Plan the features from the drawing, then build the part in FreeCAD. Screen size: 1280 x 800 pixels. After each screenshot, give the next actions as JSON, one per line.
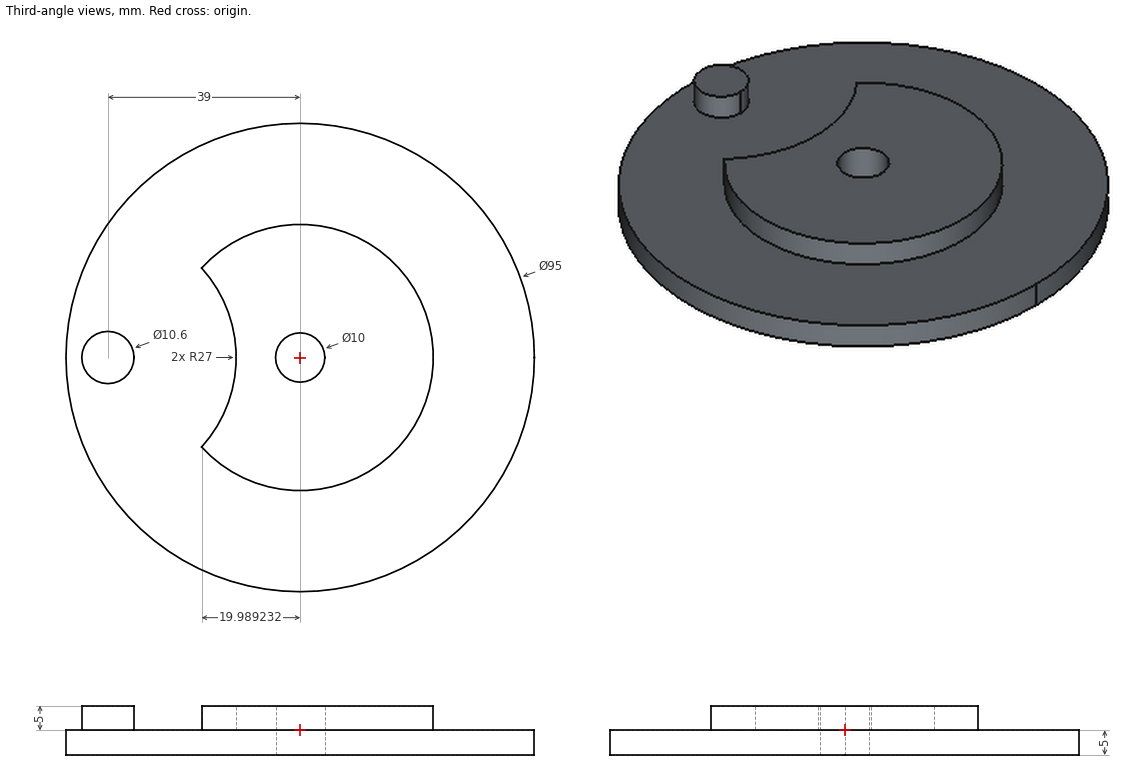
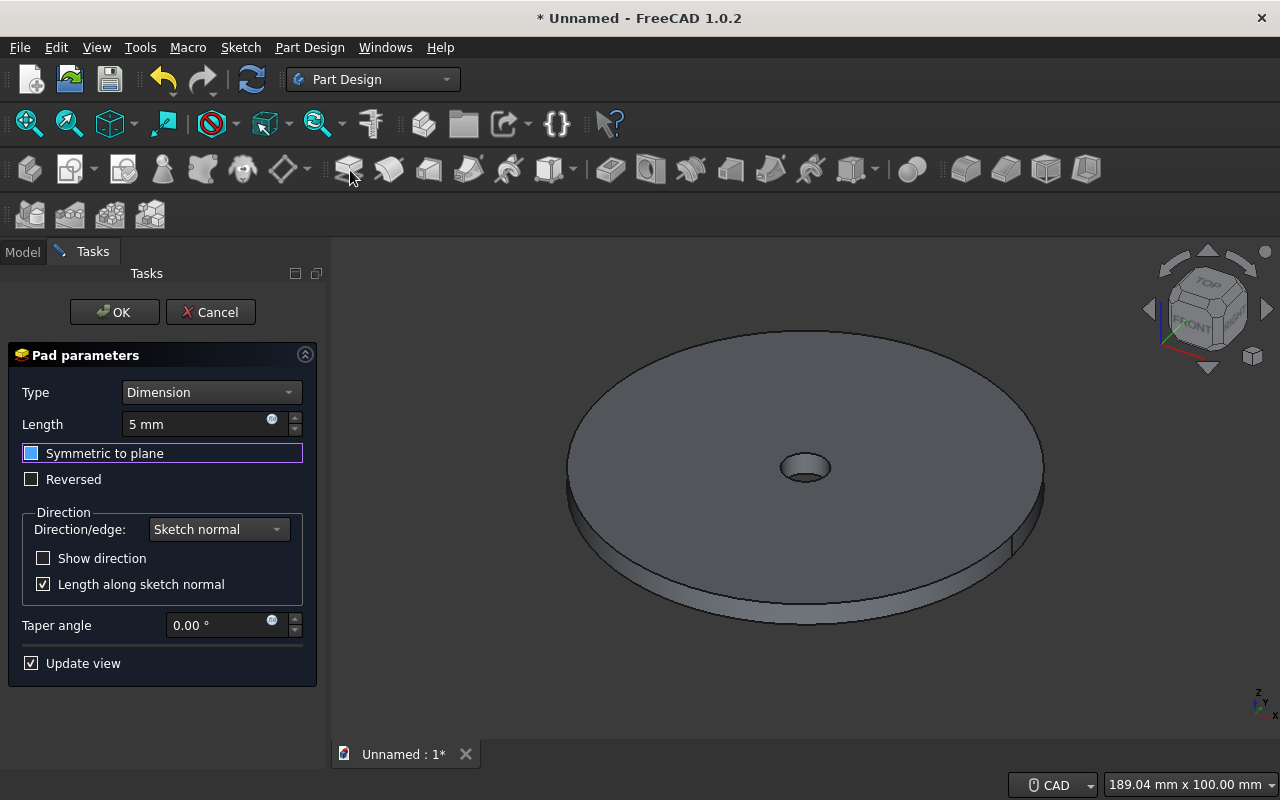
{"action": "left_click", "coordinate": [30, 479]}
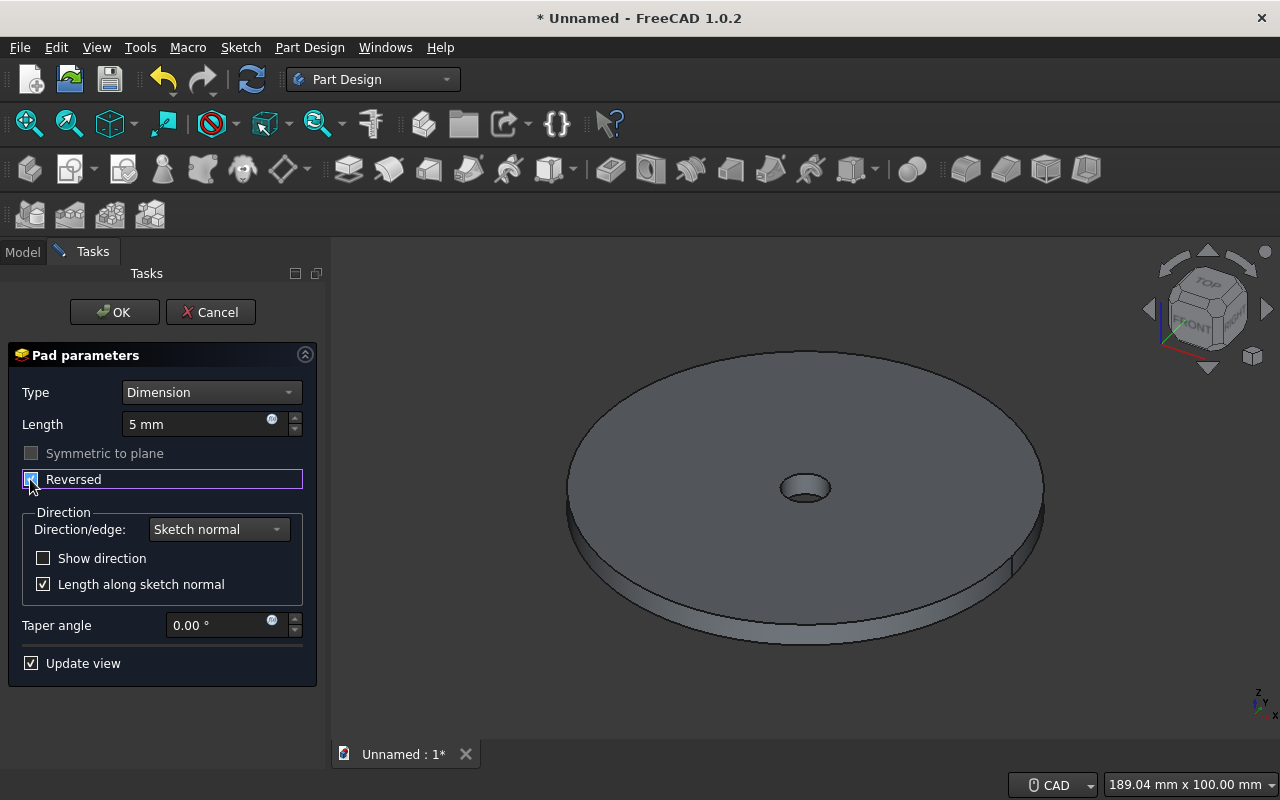
{"action": "left_click", "coordinate": [115, 312]}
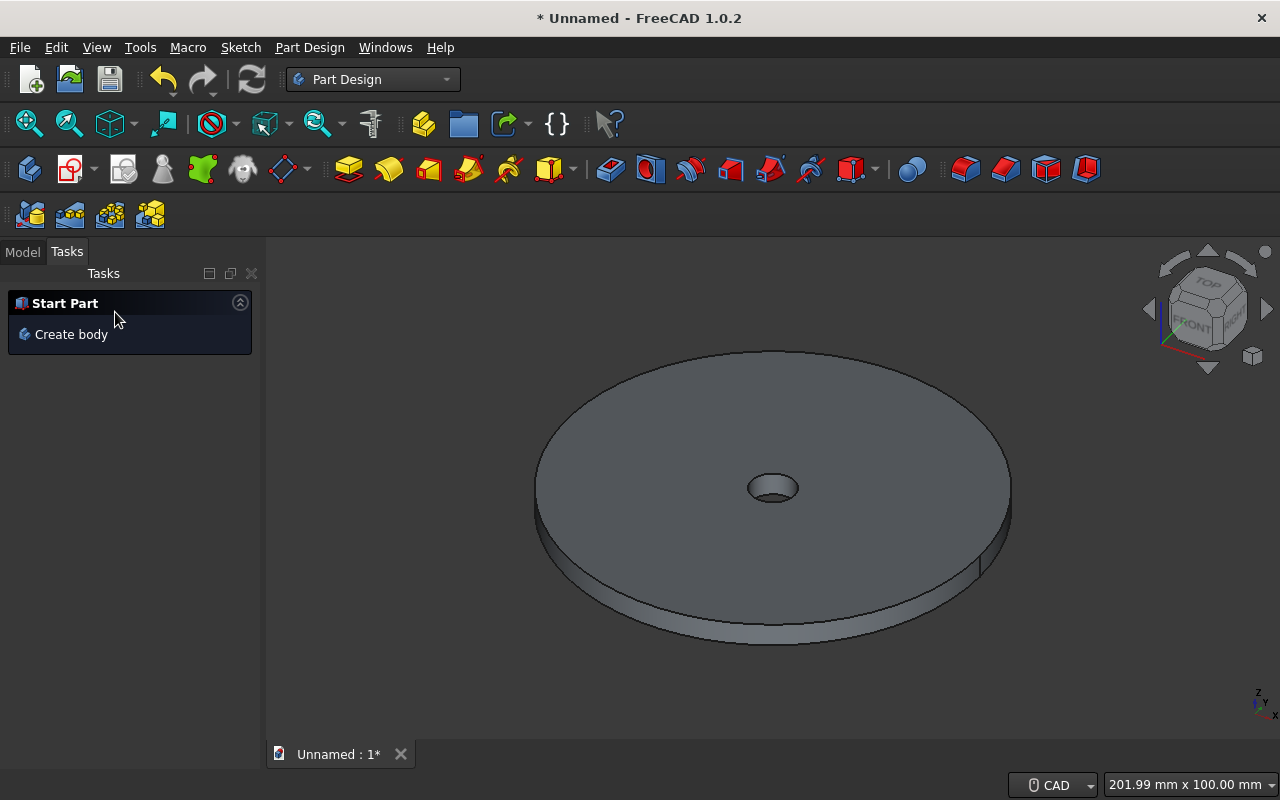
{"action": "left_click", "coordinate": [23, 251]}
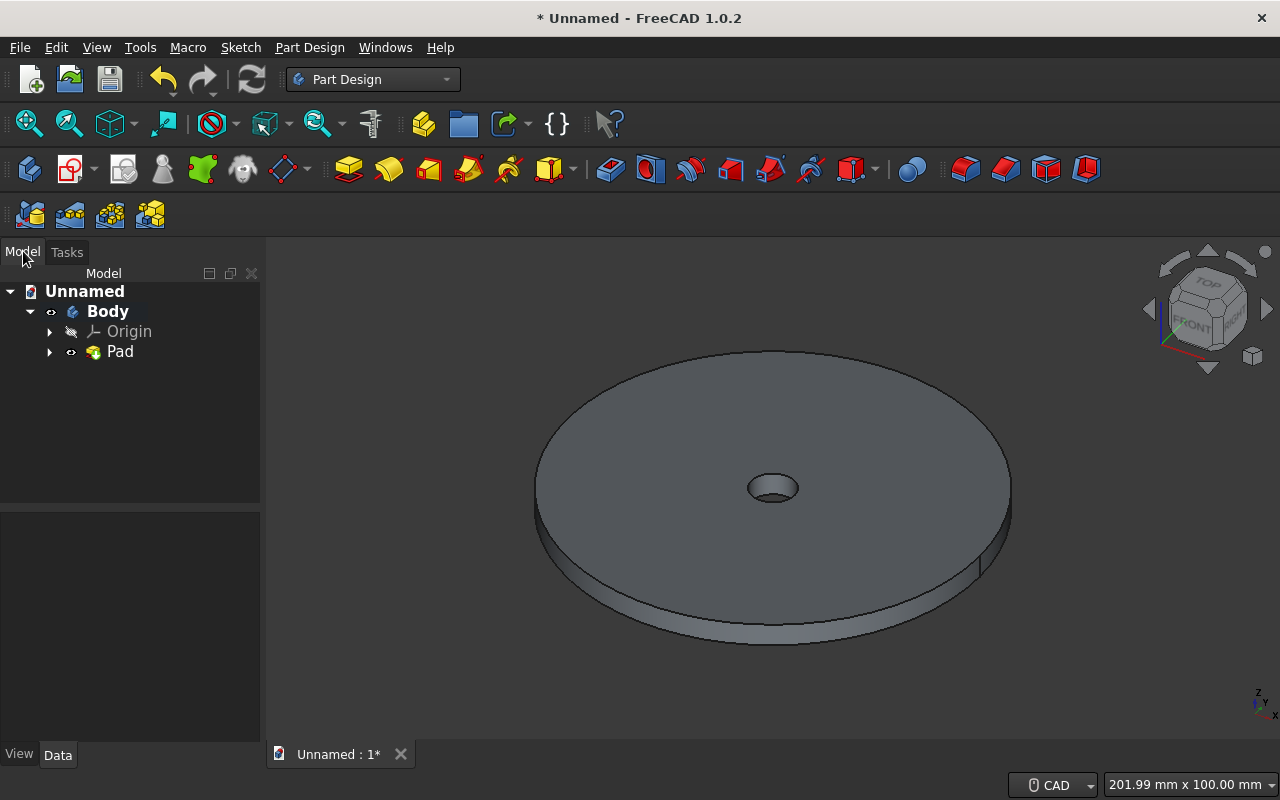
{"action": "left_click", "coordinate": [50, 332]}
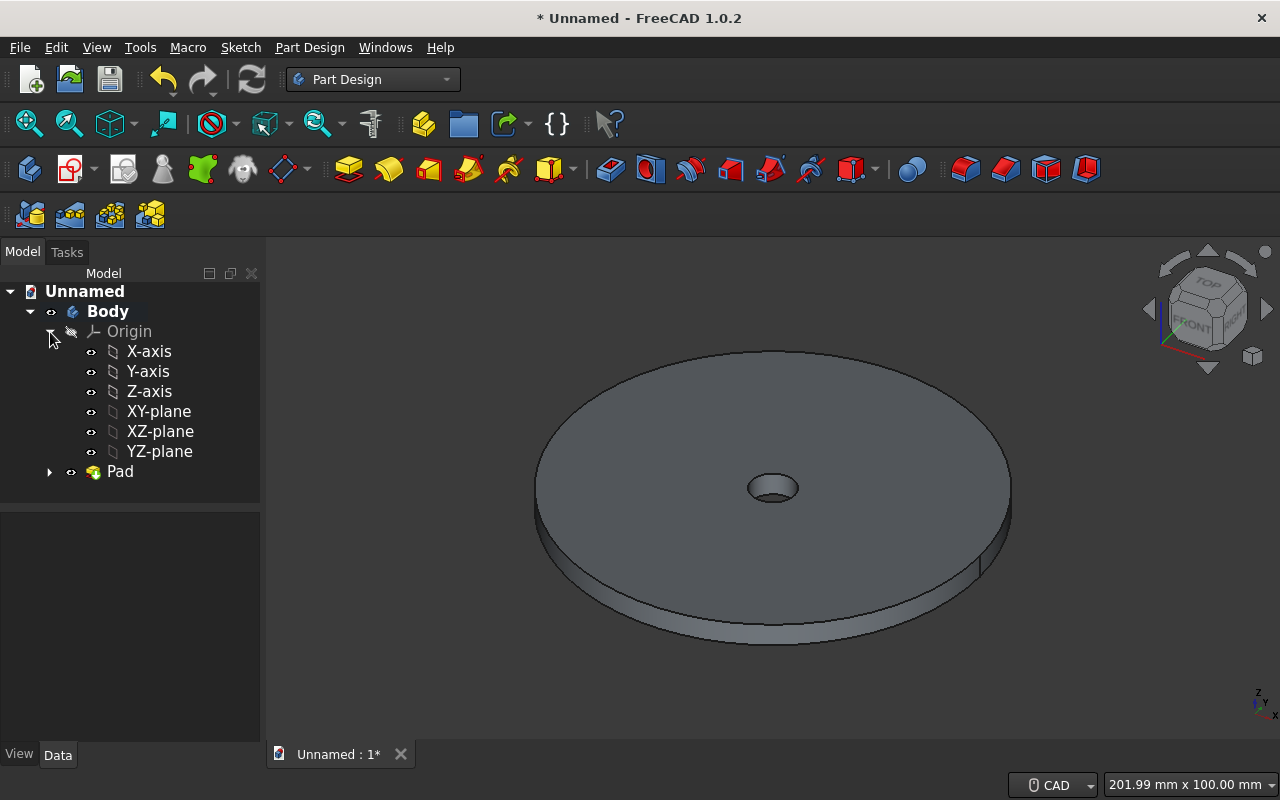
{"action": "left_click", "coordinate": [136, 412]}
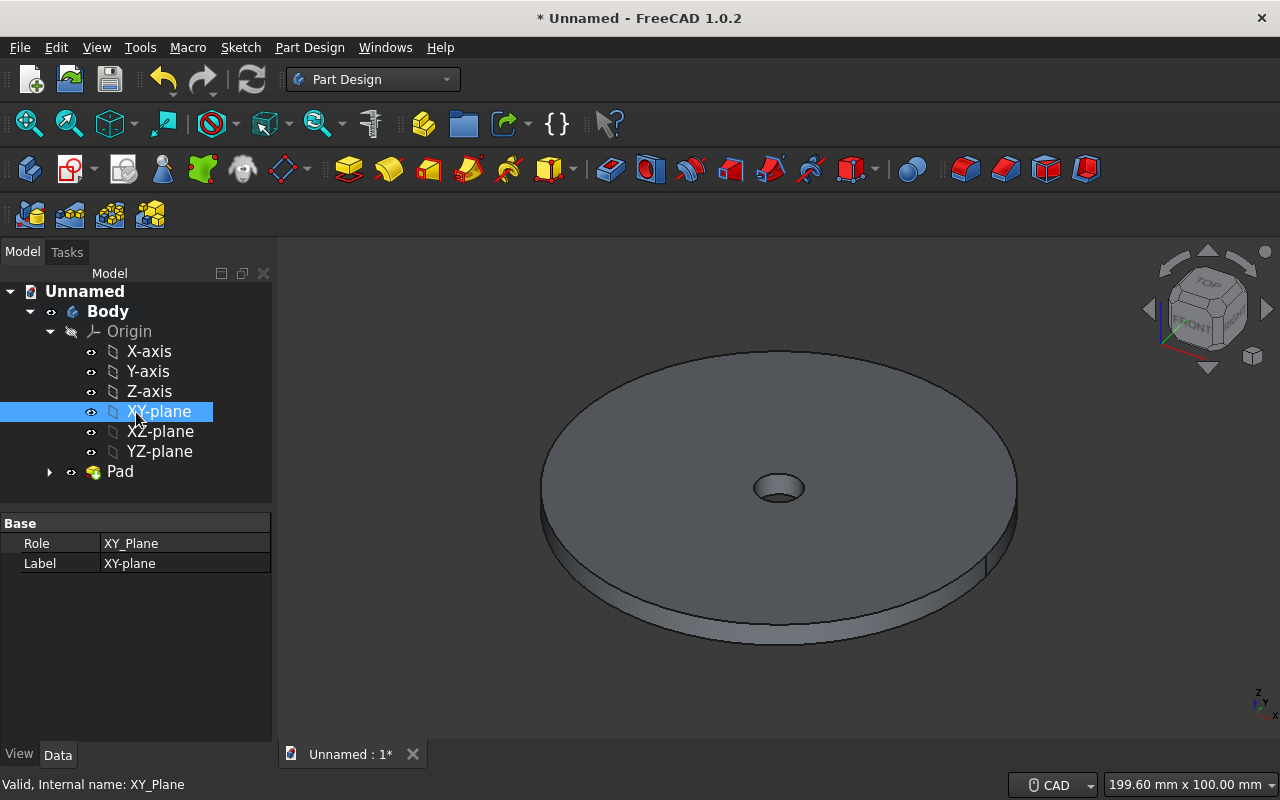
{"action": "left_click", "coordinate": [284, 170]}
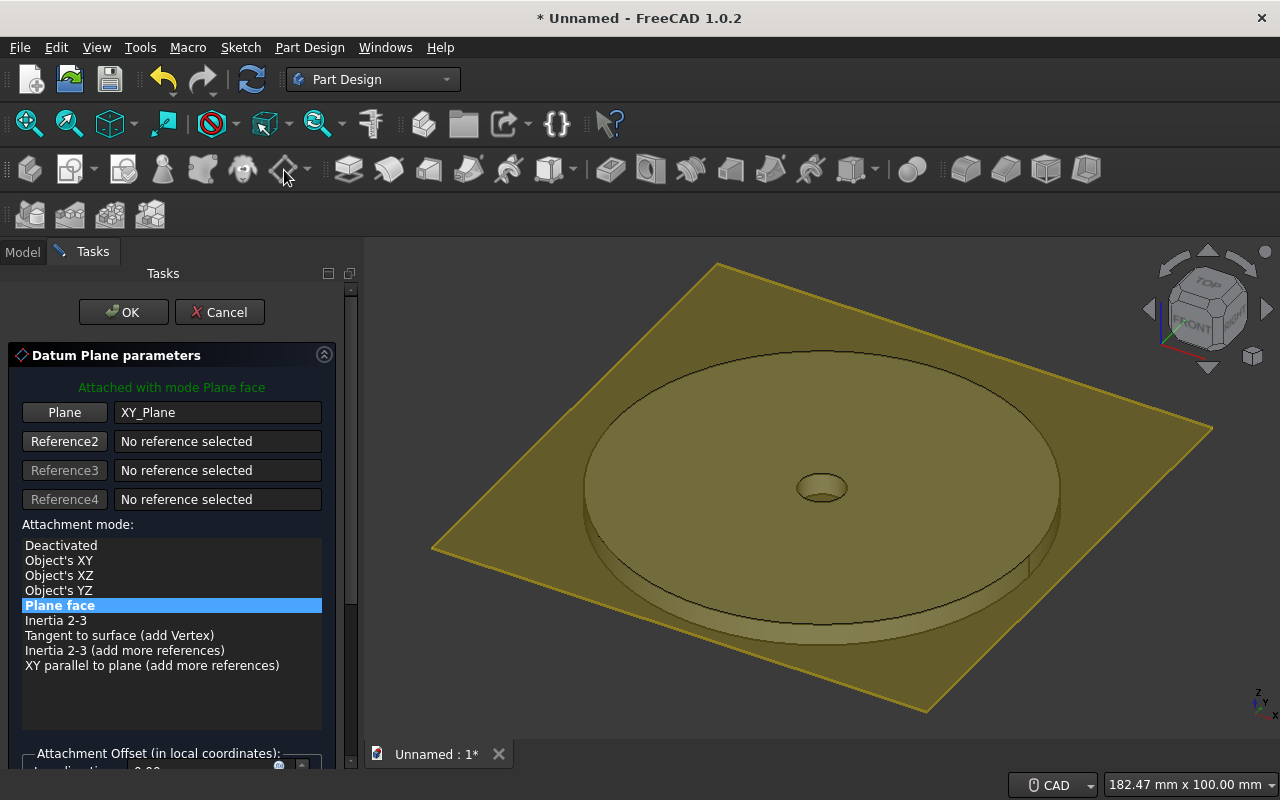
{"action": "scroll", "coordinate": [351, 526], "scroll_direction": "down", "scroll_amount": 3}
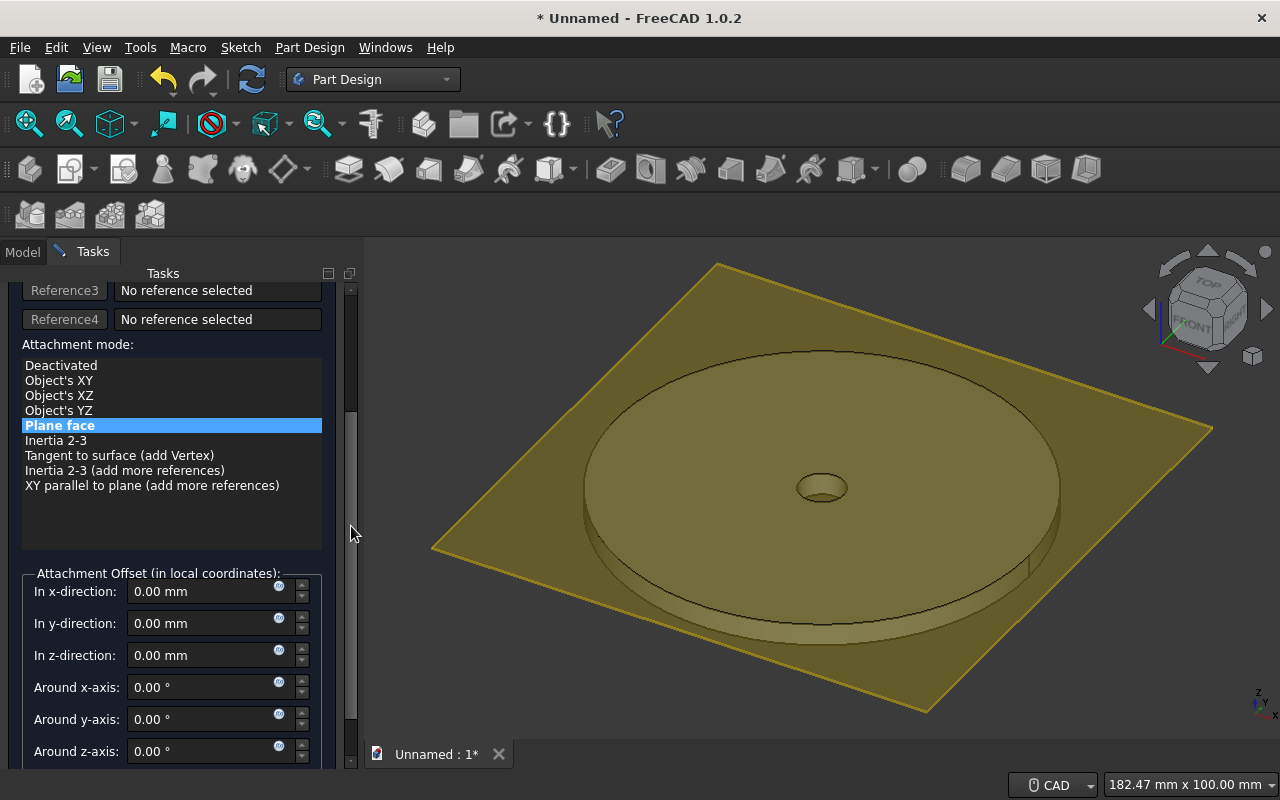
{"action": "triple_click", "coordinate": [210, 655]}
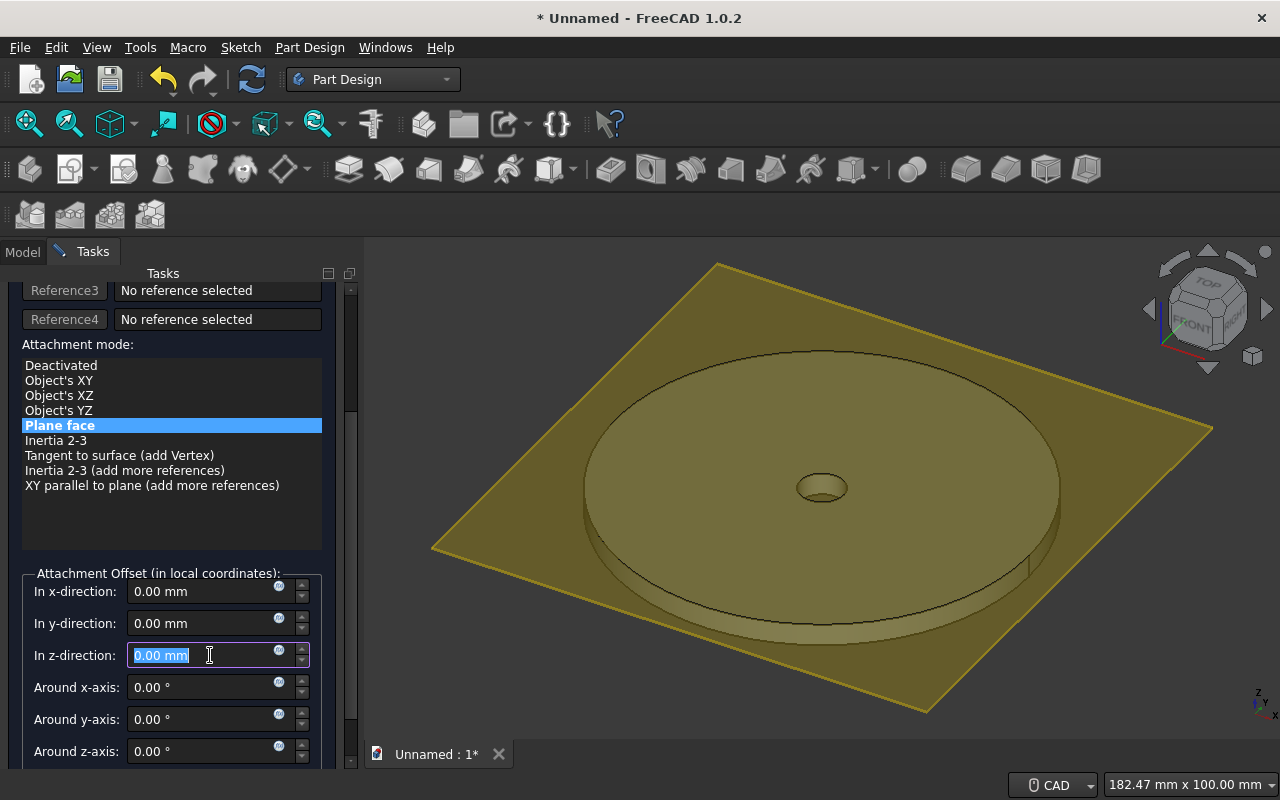
{"action": "type", "text": "5"}
{"action": "key", "text": "Tab"}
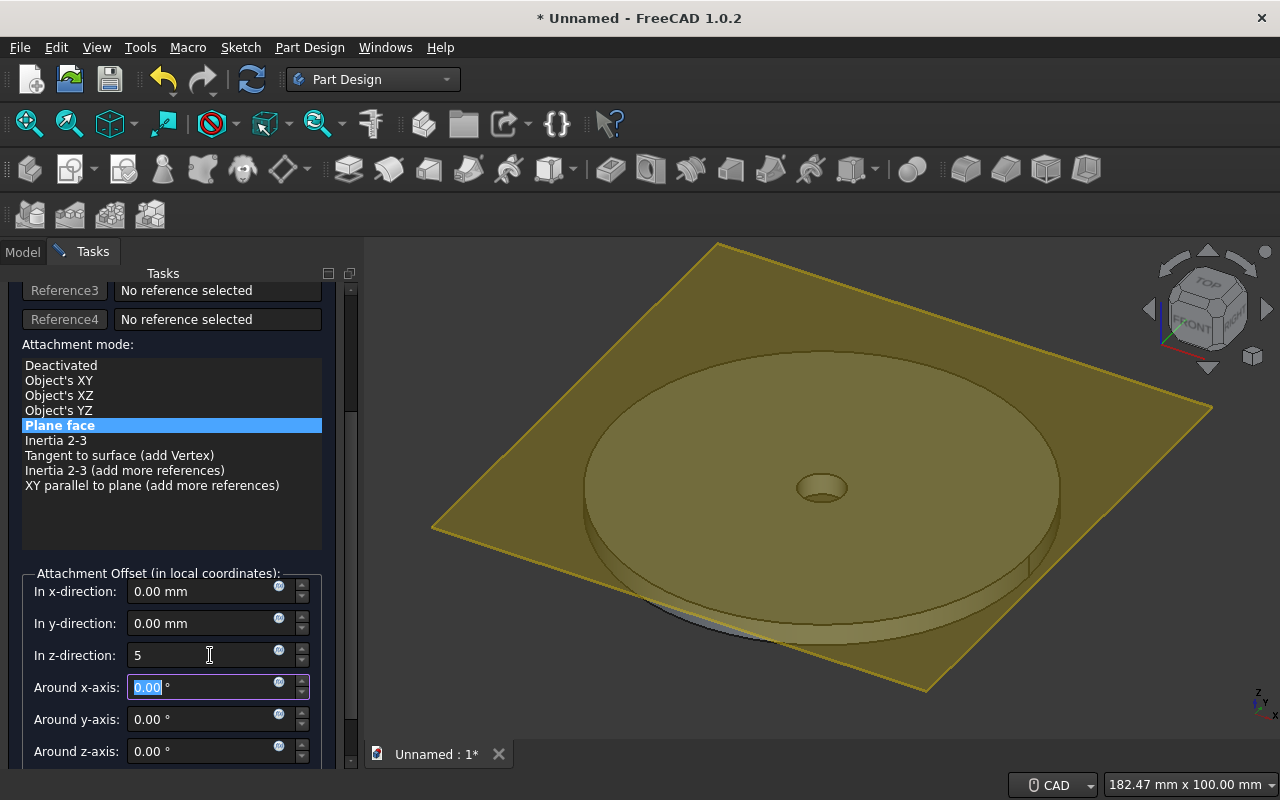
{"action": "scroll", "coordinate": [351, 526], "scroll_direction": "up", "scroll_amount": 4}